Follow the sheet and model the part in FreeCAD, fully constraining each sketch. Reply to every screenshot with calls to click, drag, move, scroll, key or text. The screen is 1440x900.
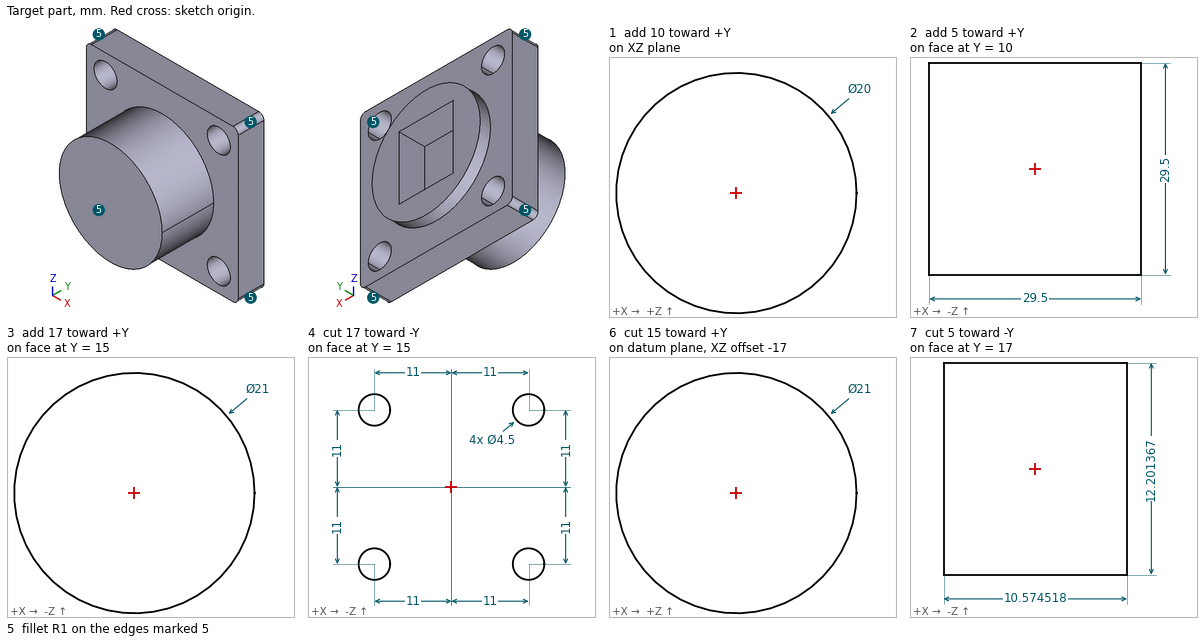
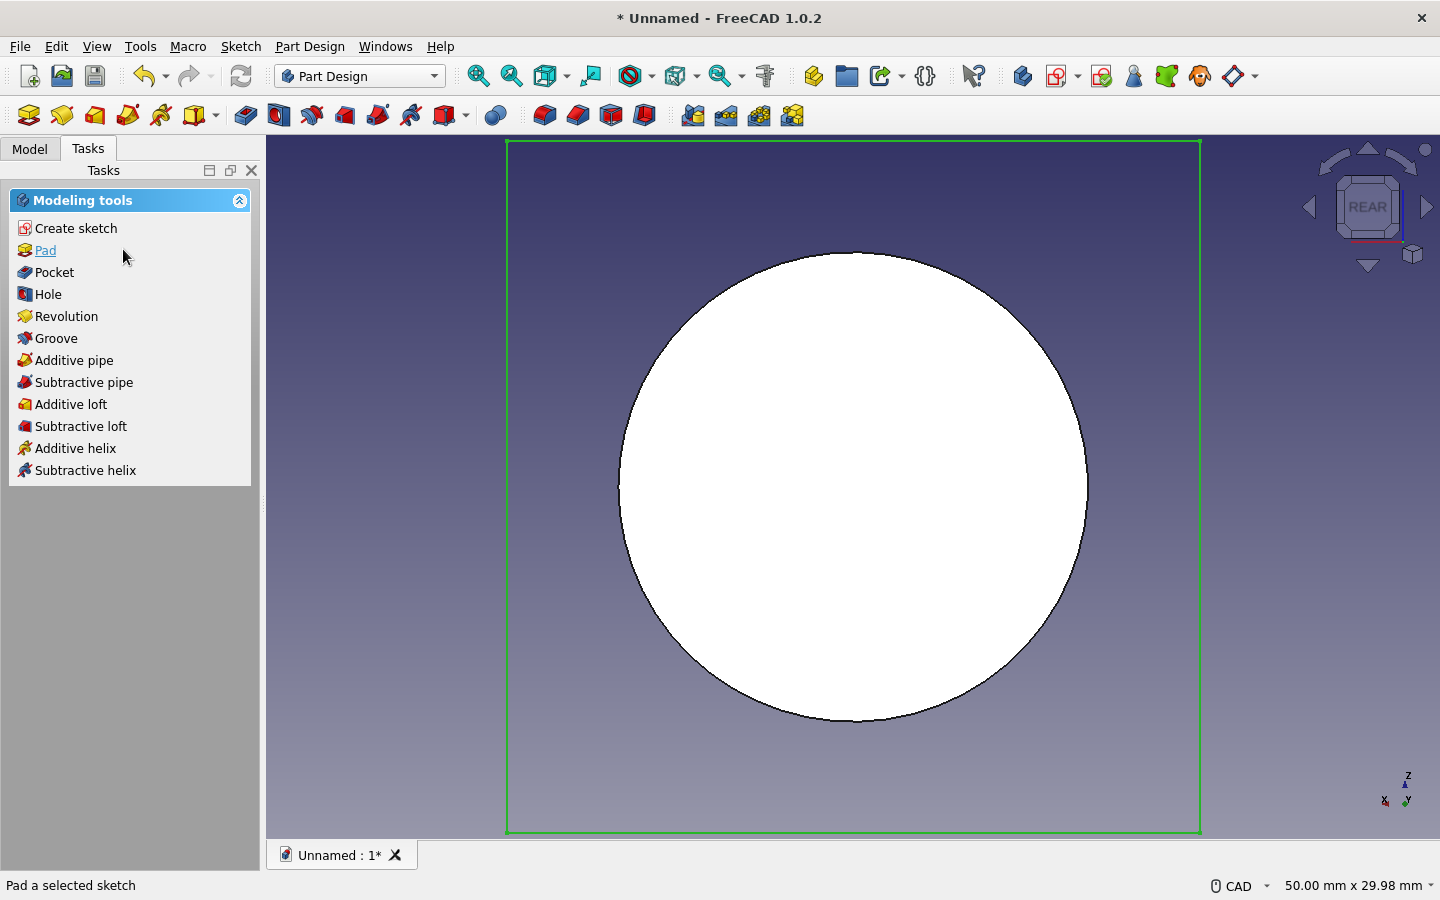
click(29, 116)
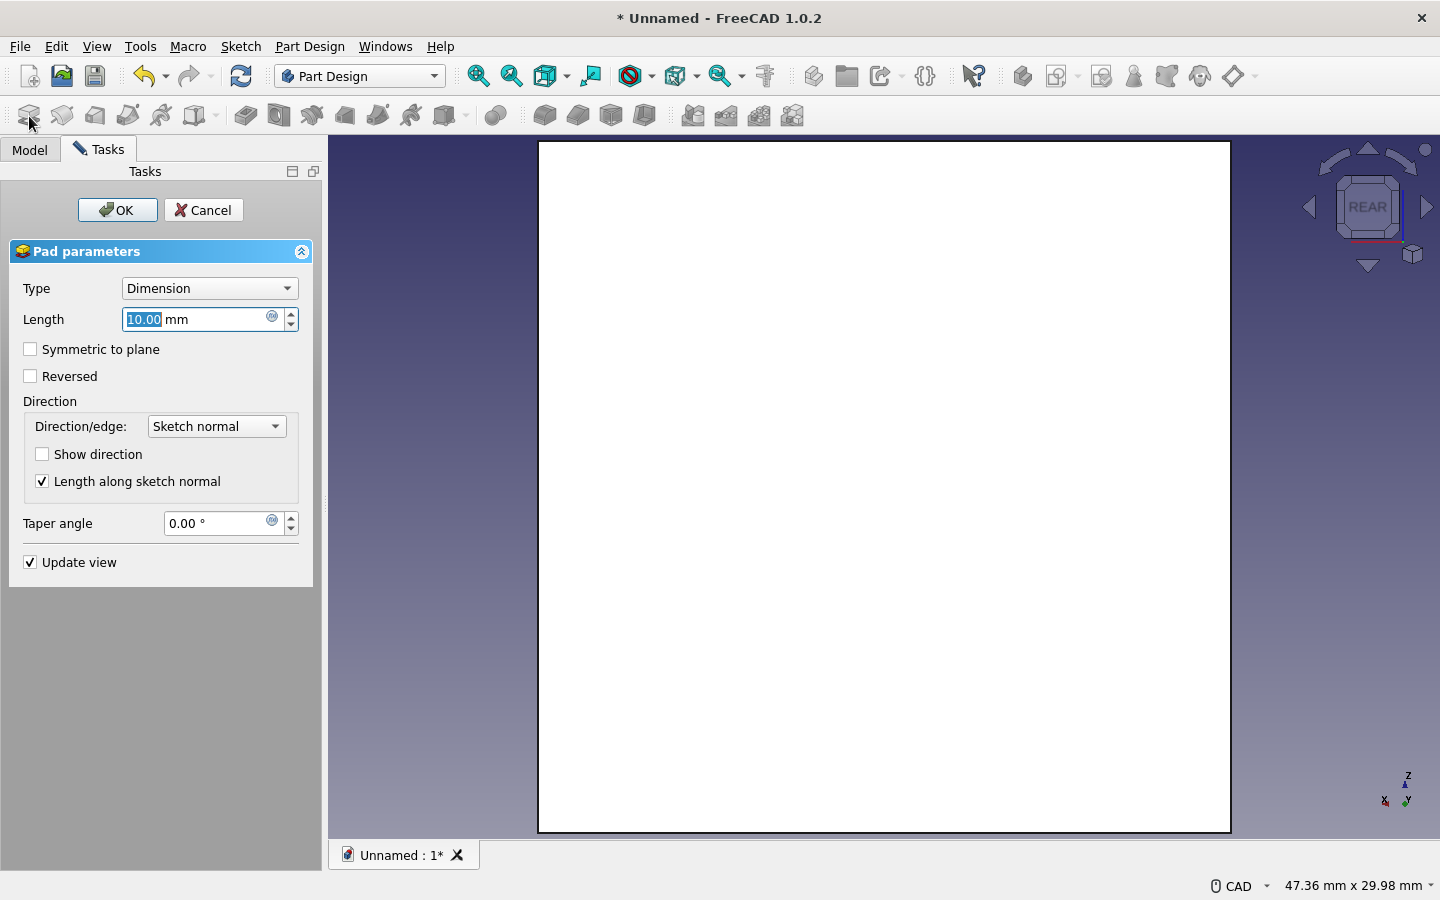
text(5)
key(Tab)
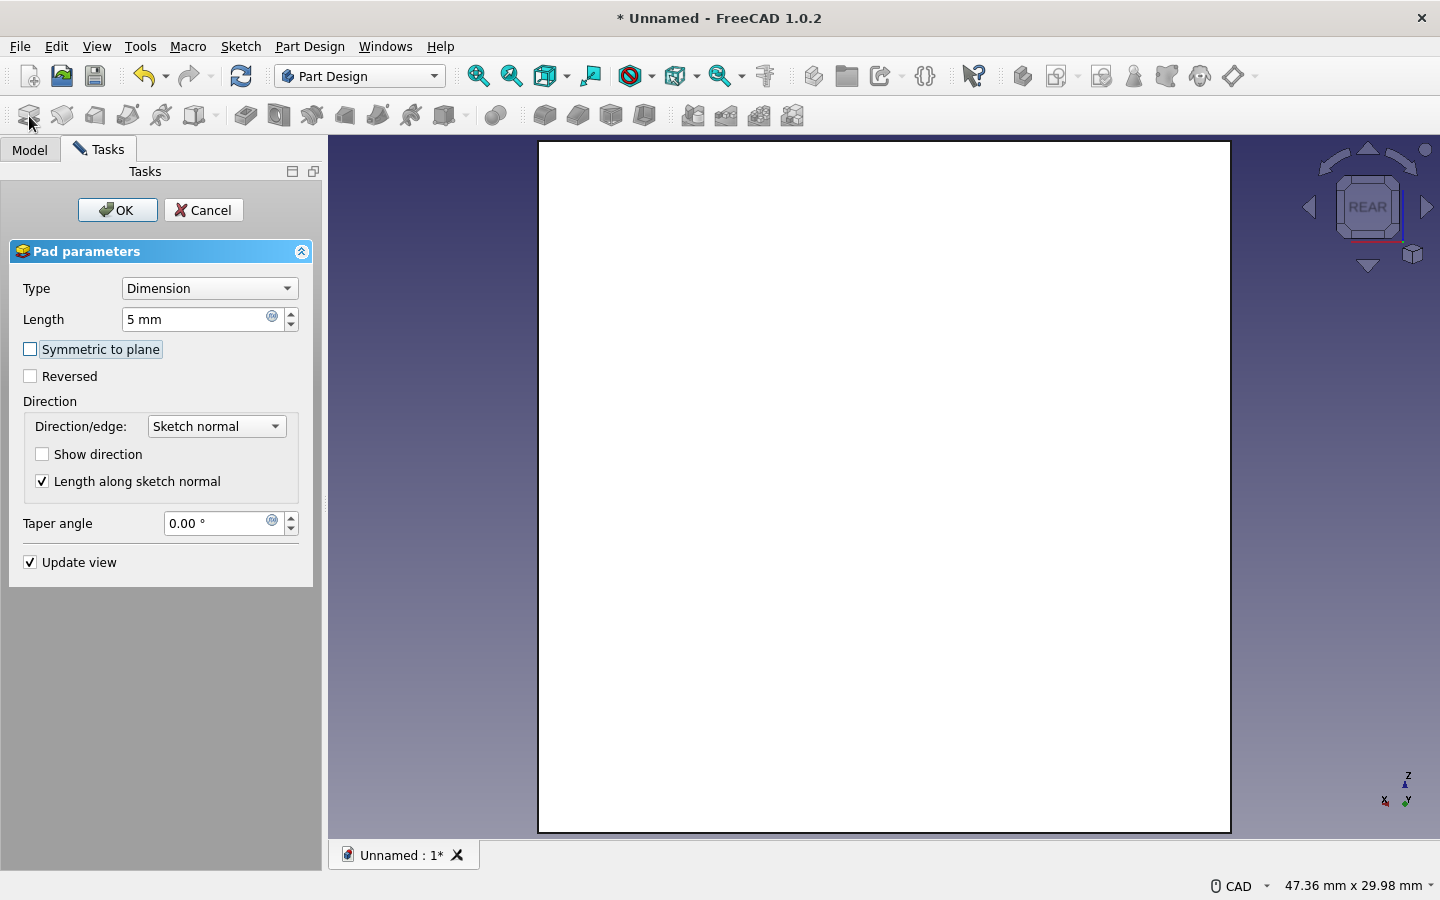
click(118, 210)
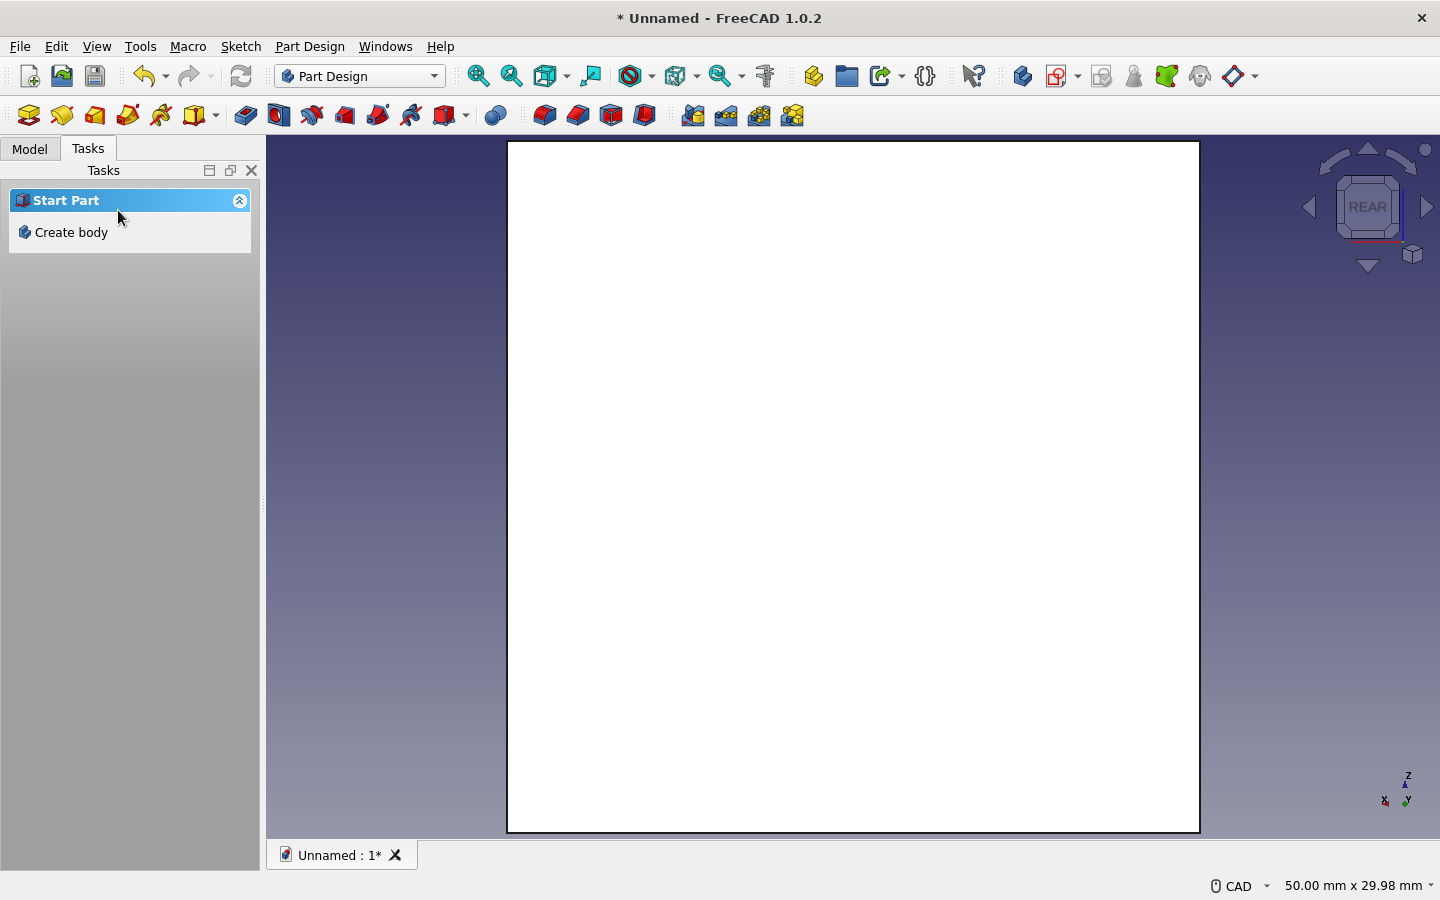
click(853, 486)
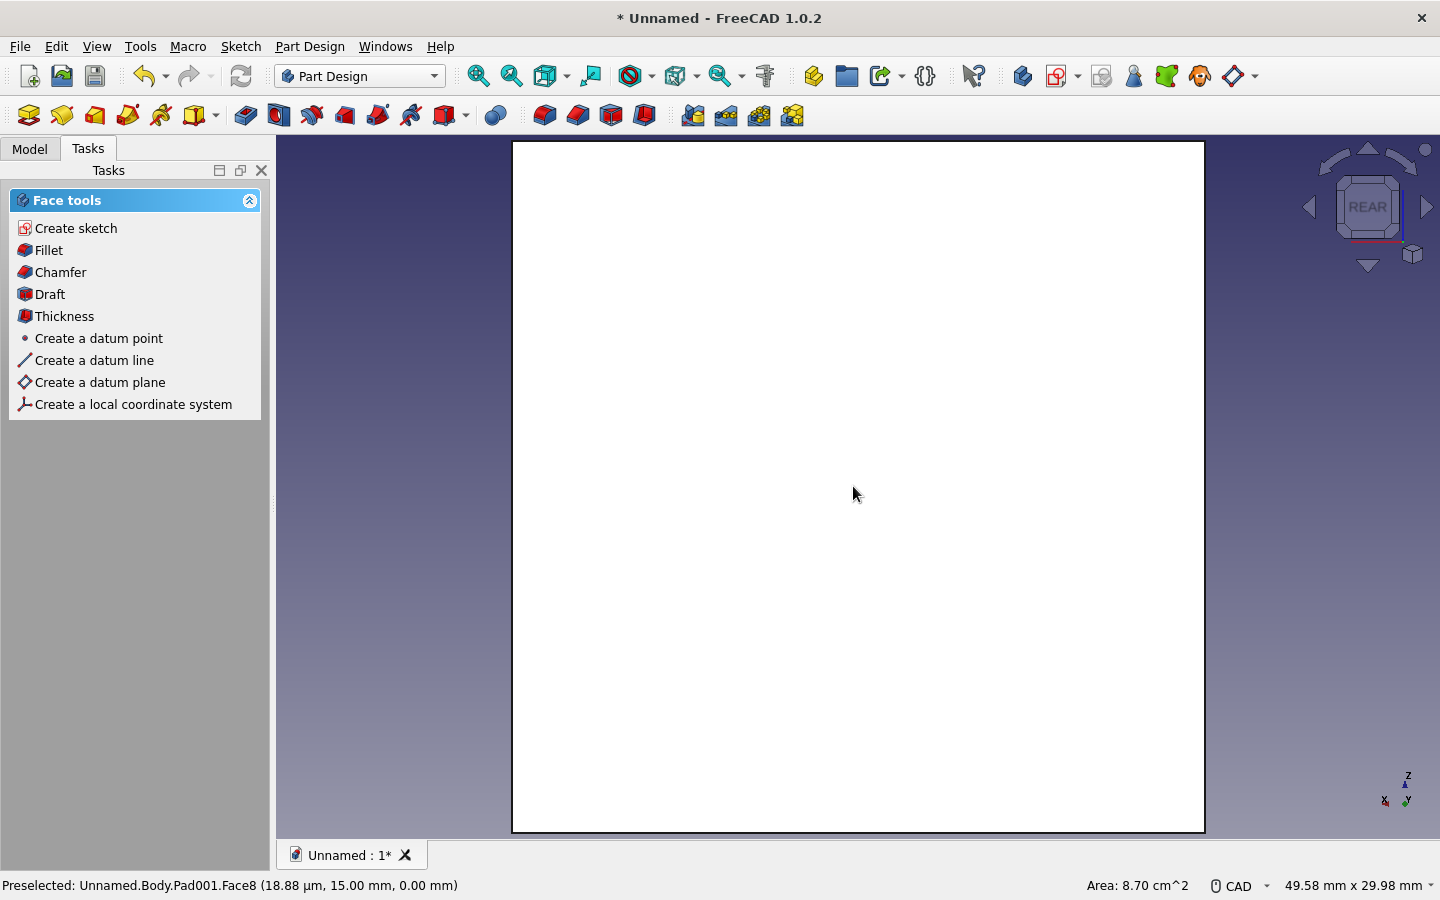
click(1056, 76)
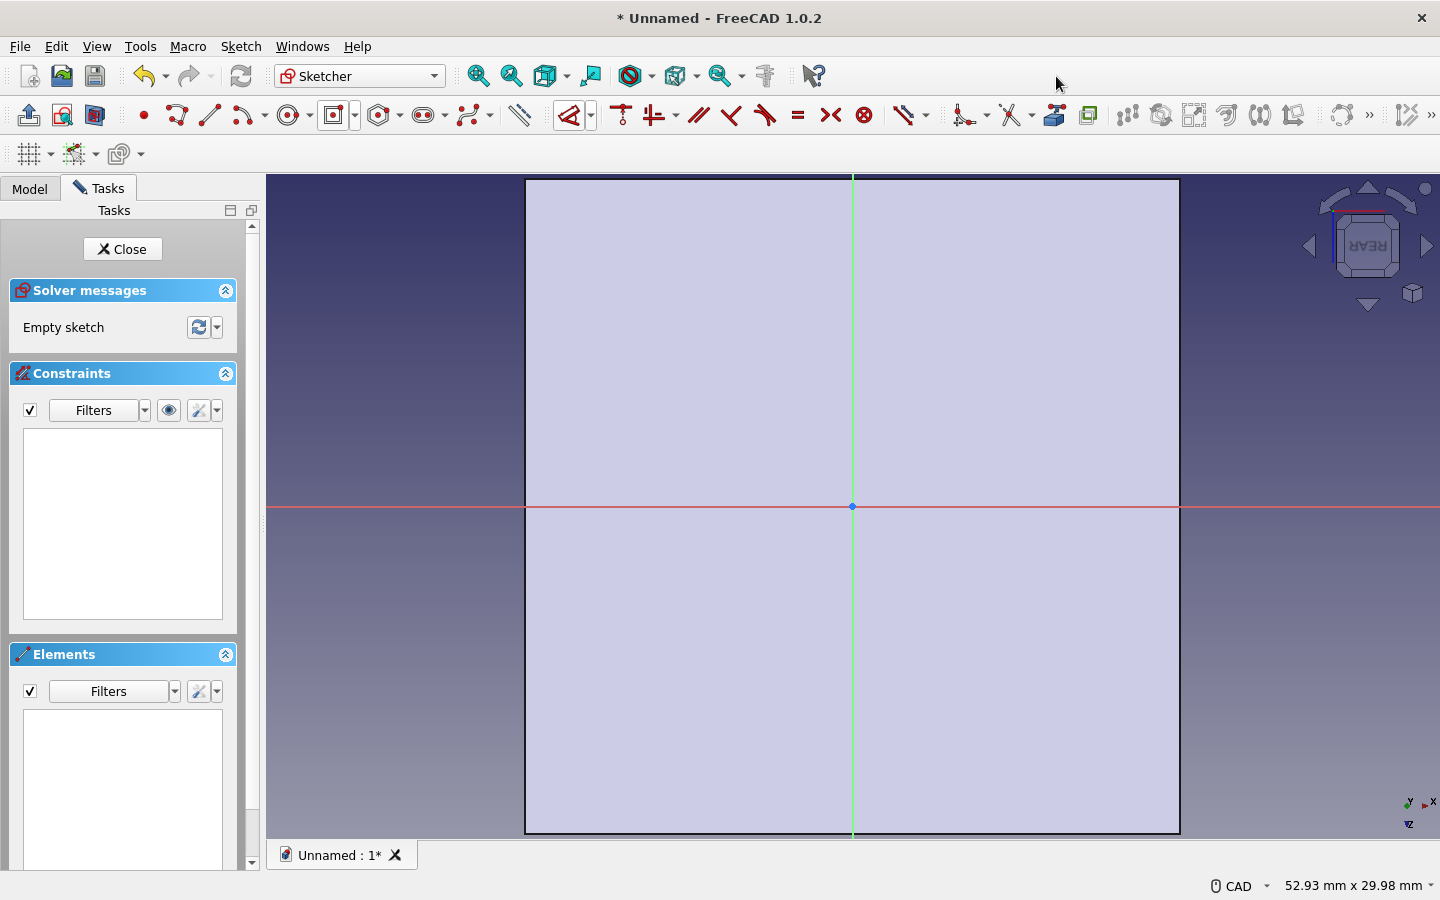
click(288, 116)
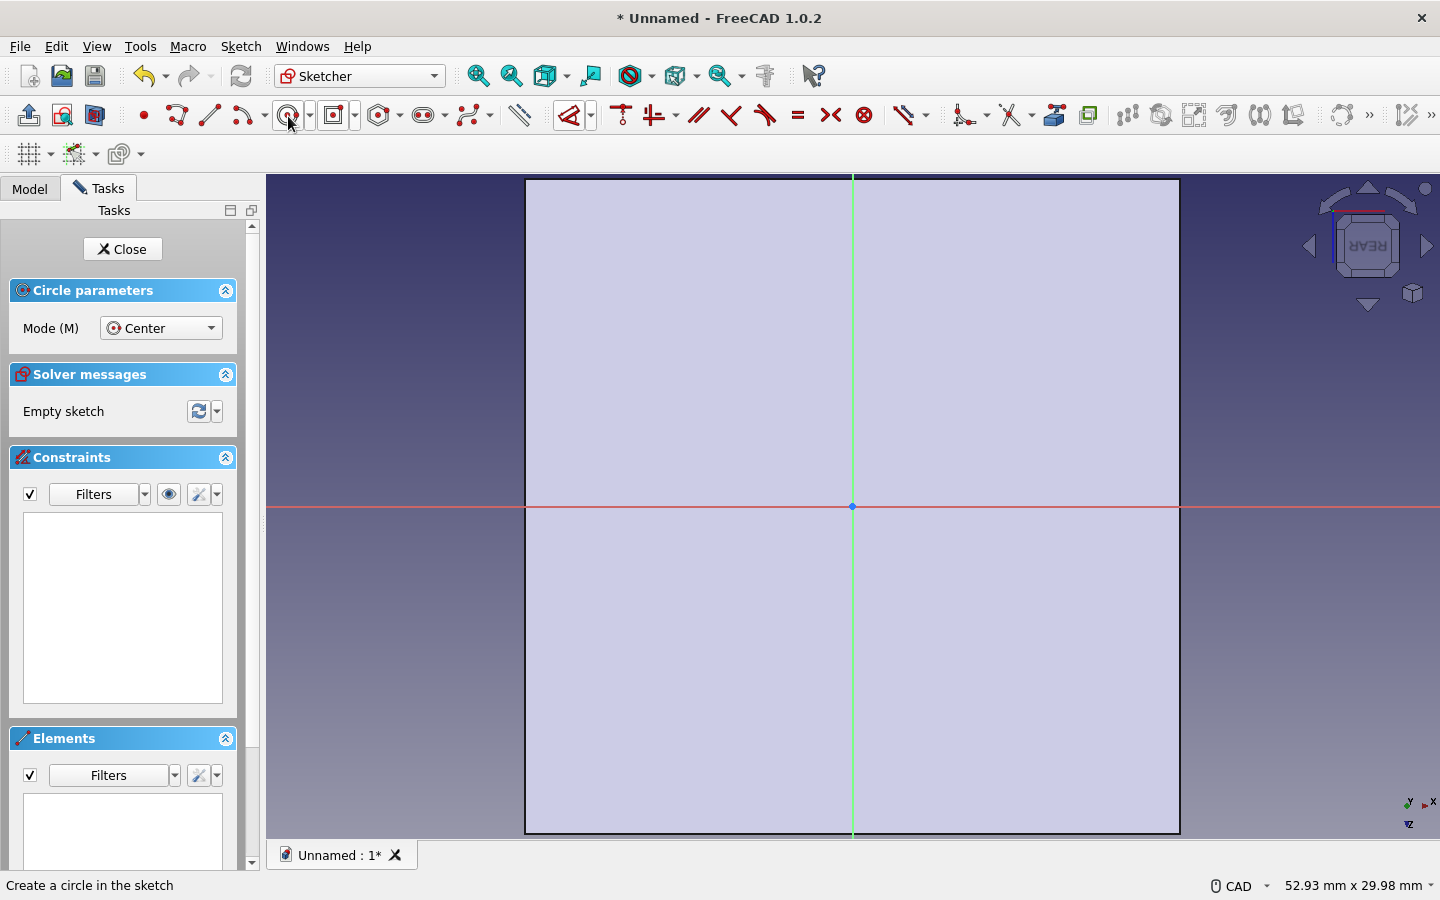
click(853, 506)
click(1017, 342)
key(Escape)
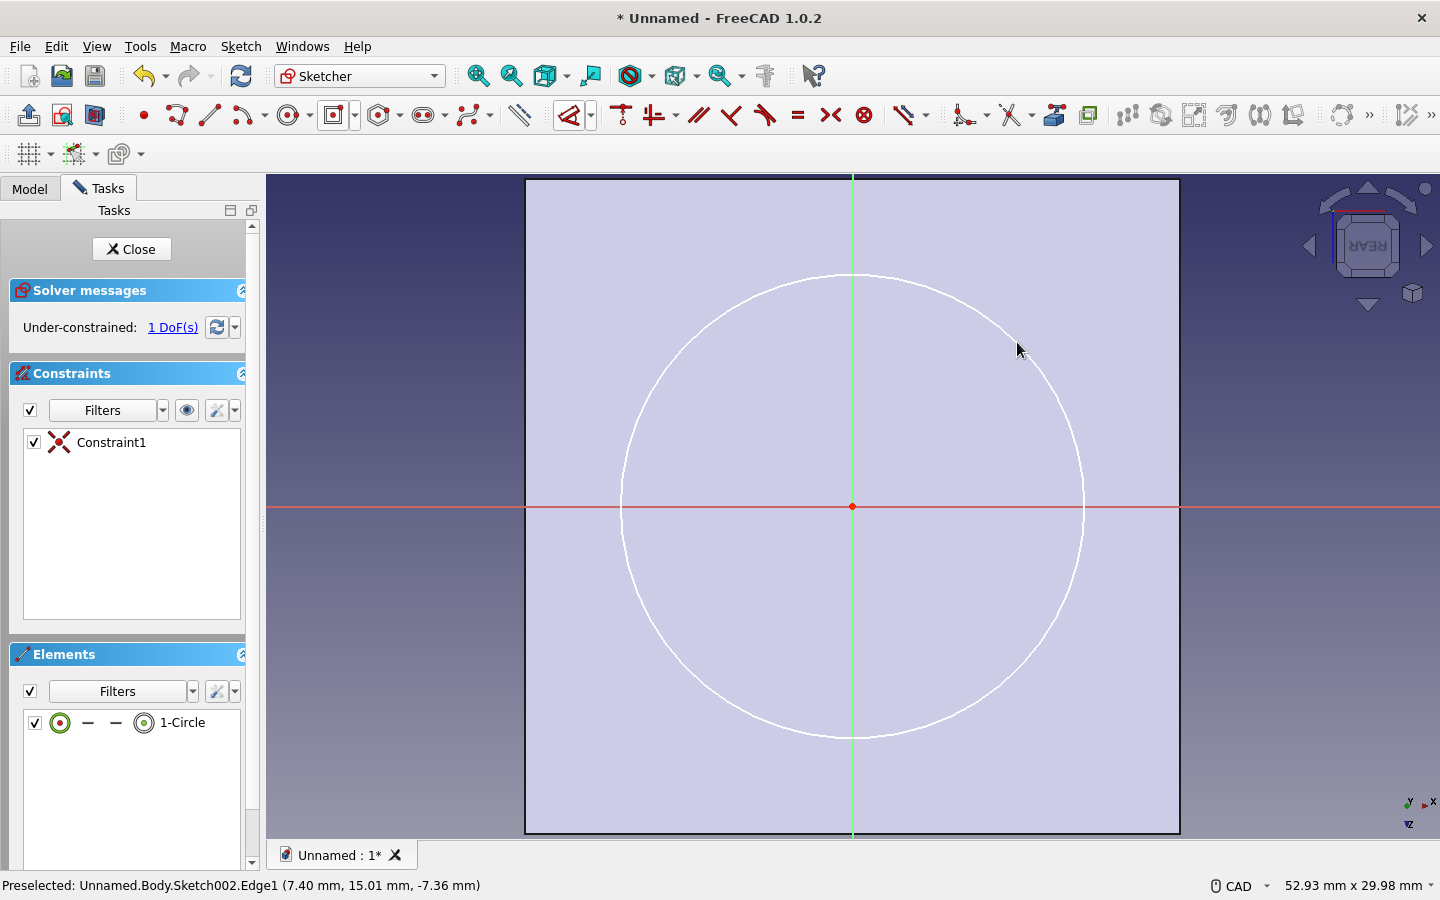
click(1016, 342)